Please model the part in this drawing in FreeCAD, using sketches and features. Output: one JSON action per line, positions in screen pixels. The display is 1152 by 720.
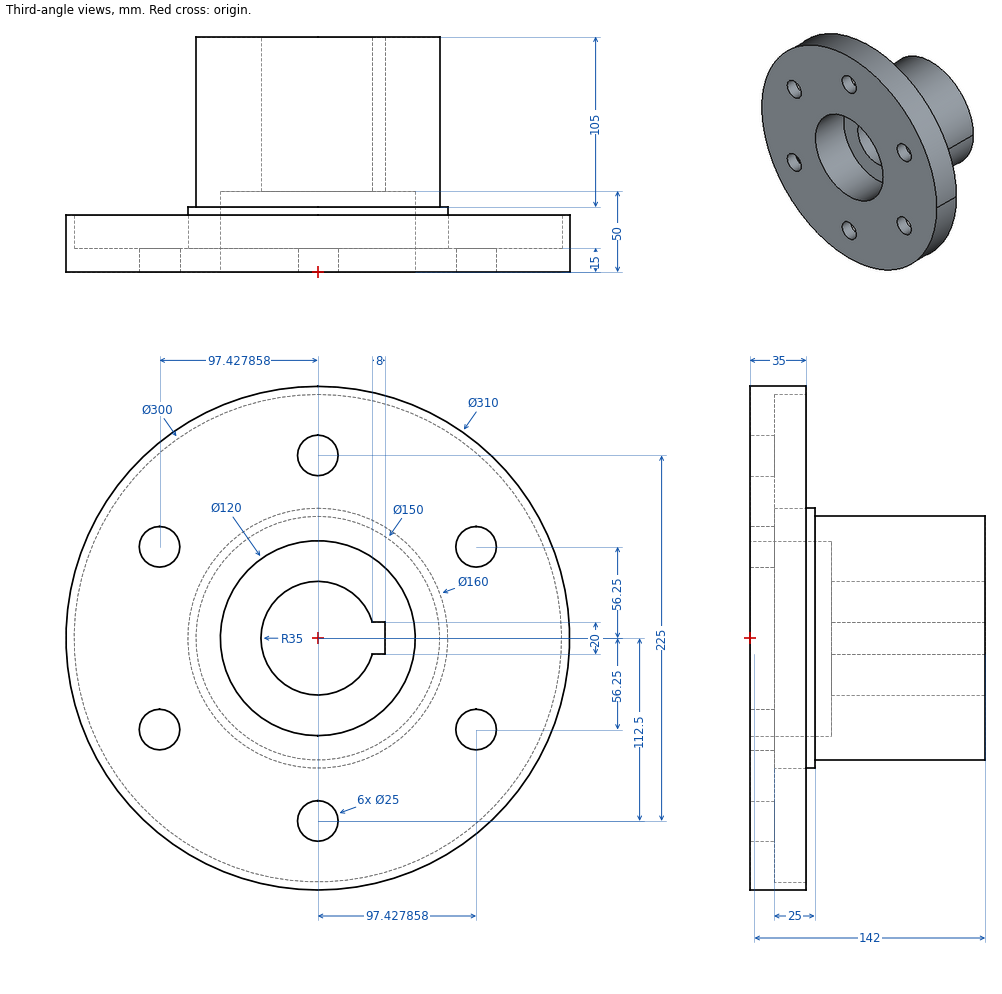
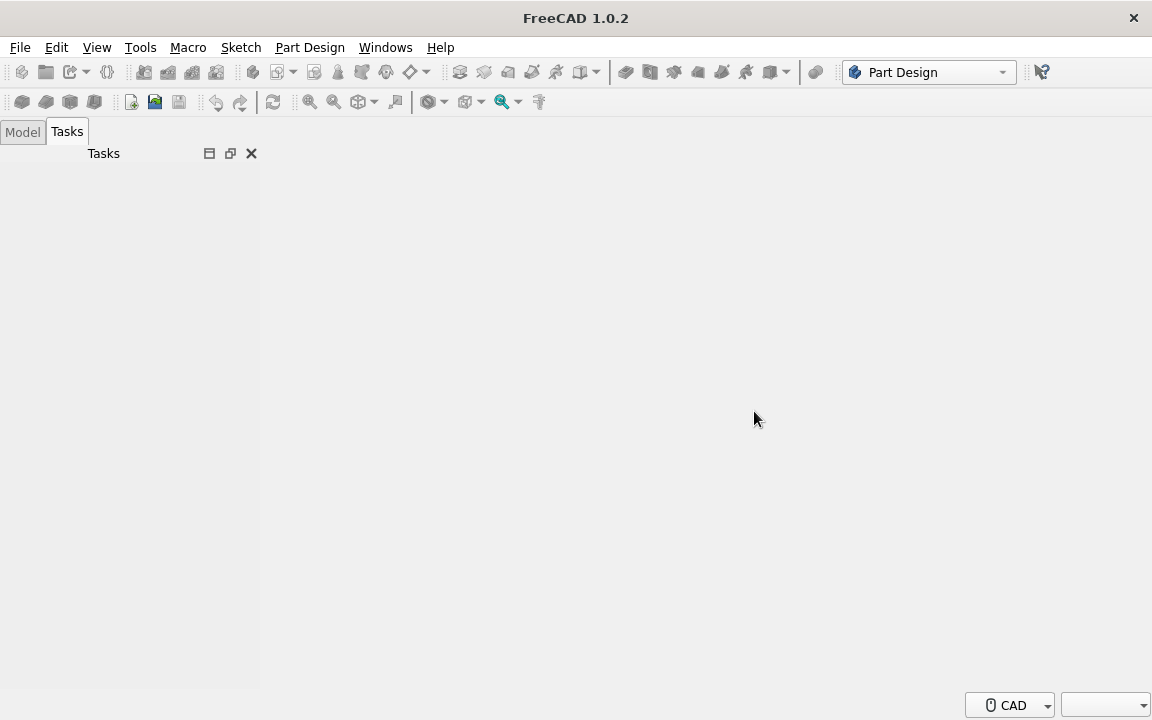
{"action": "left_click", "coordinate": [132, 102]}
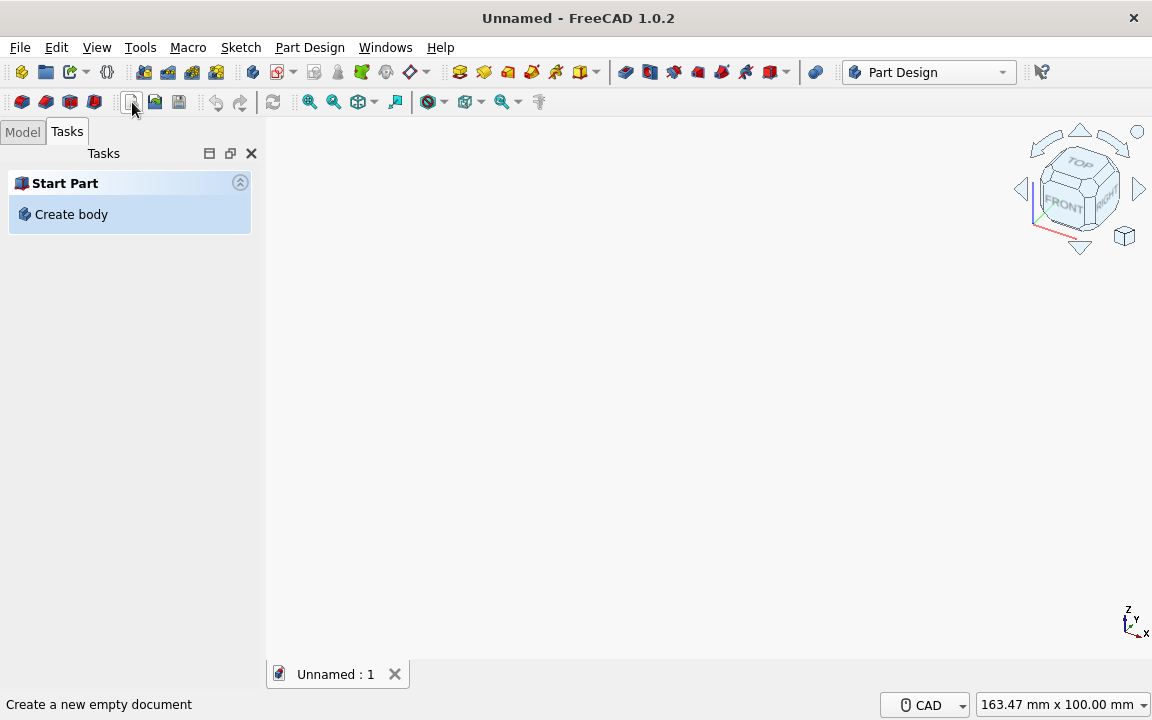
{"action": "left_click", "coordinate": [278, 72]}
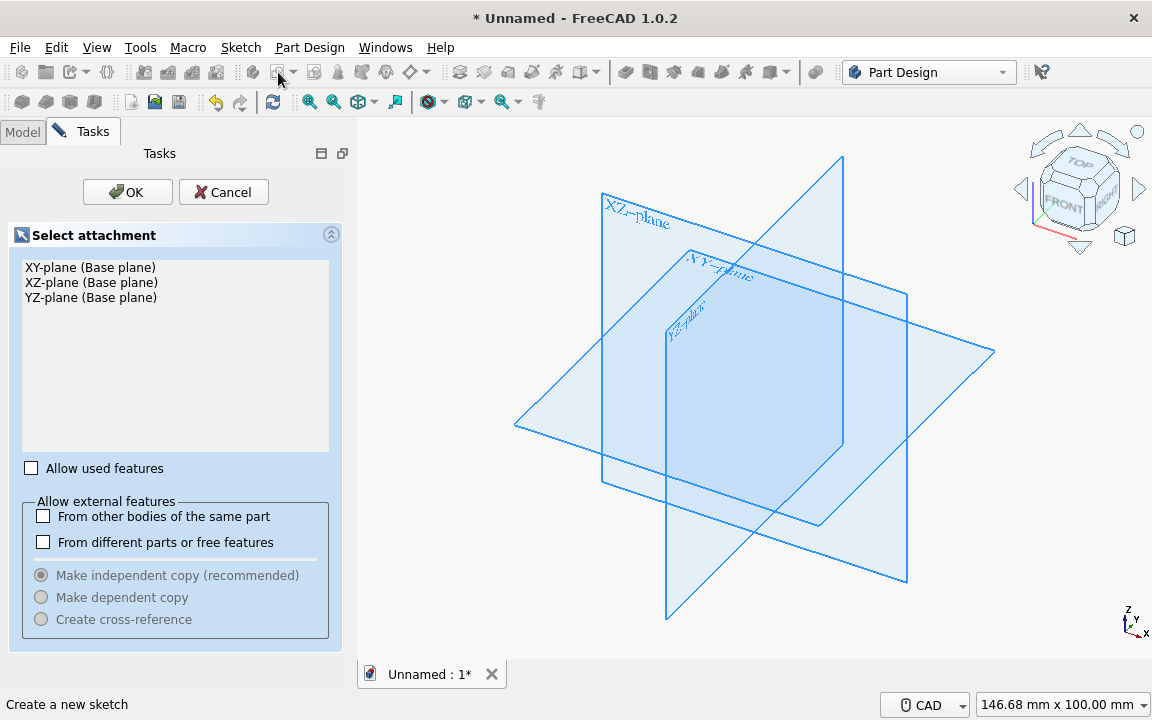
{"action": "left_click", "coordinate": [82, 282]}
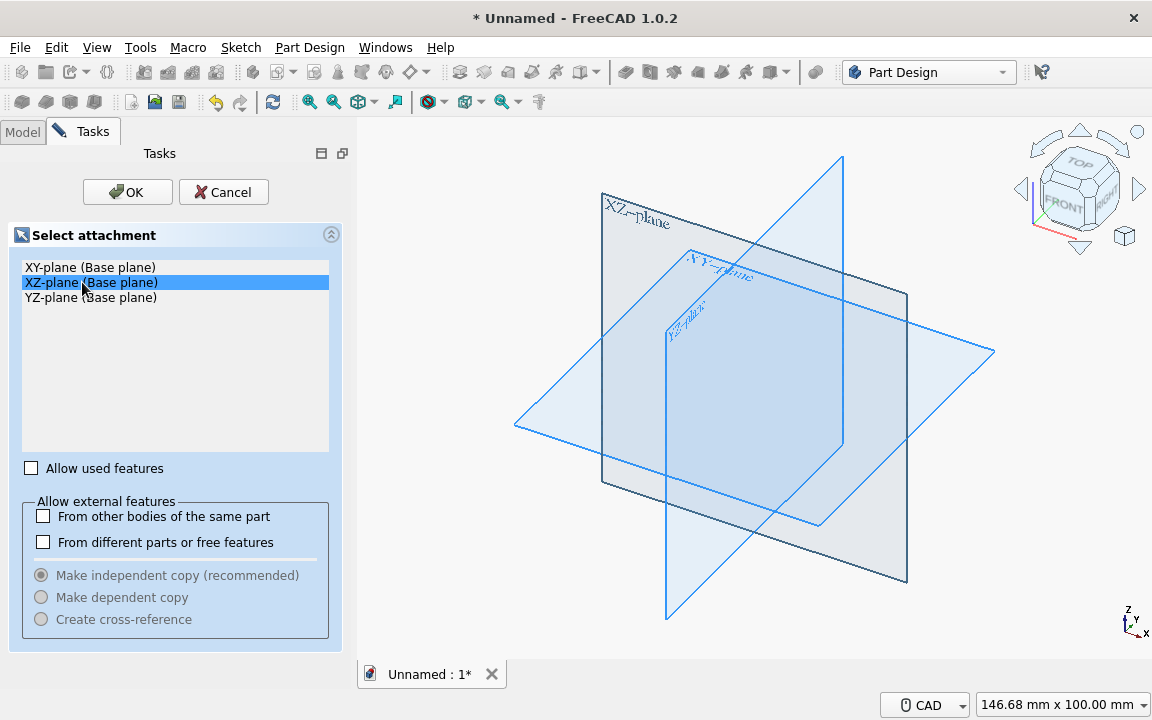
{"action": "left_click", "coordinate": [128, 192]}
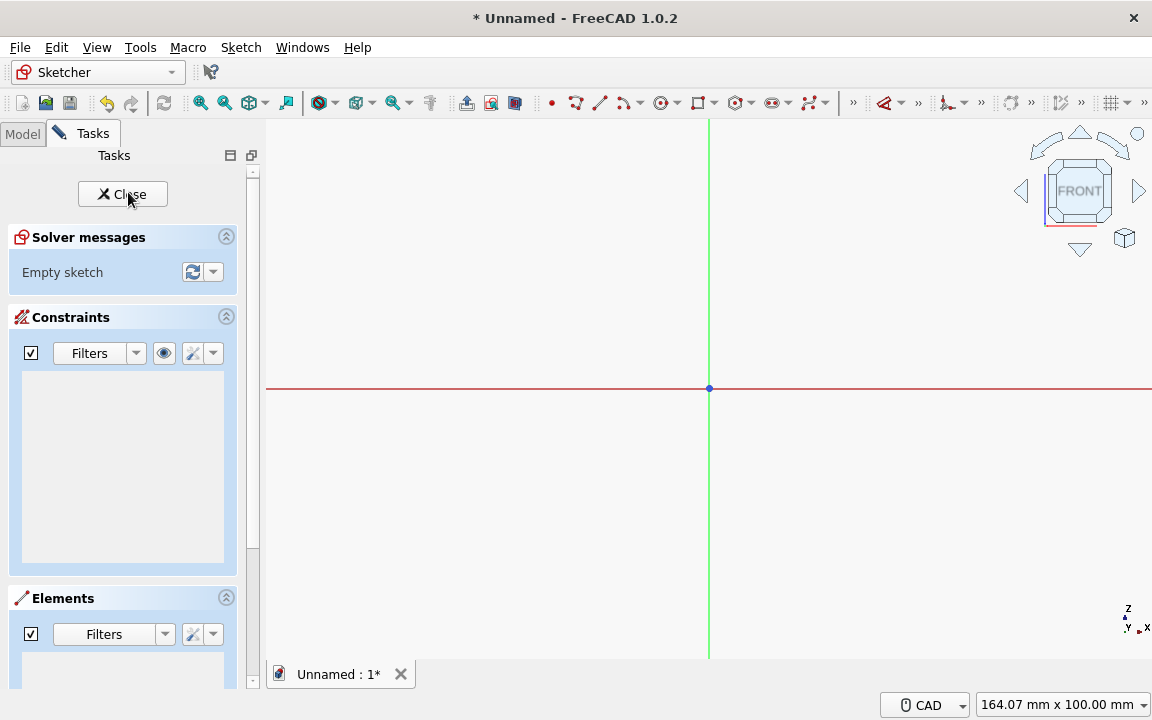
{"action": "scroll", "coordinate": [623, 389], "scroll_direction": "down", "scroll_amount": 8}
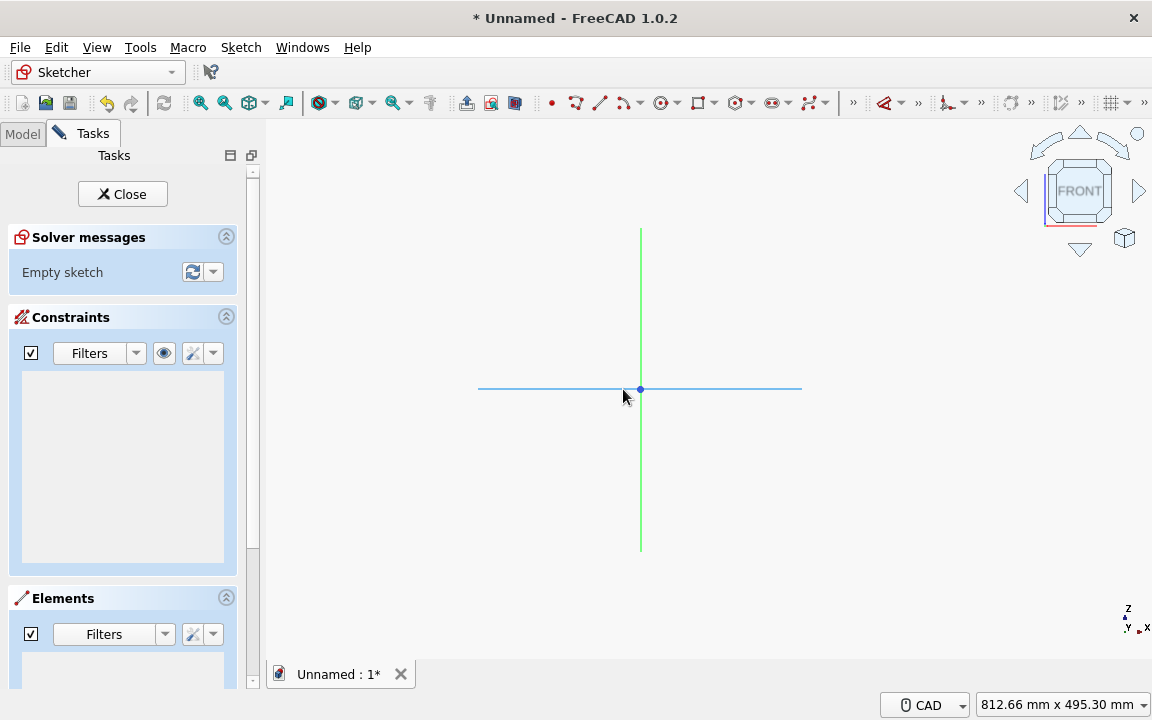
{"action": "left_click", "coordinate": [662, 104]}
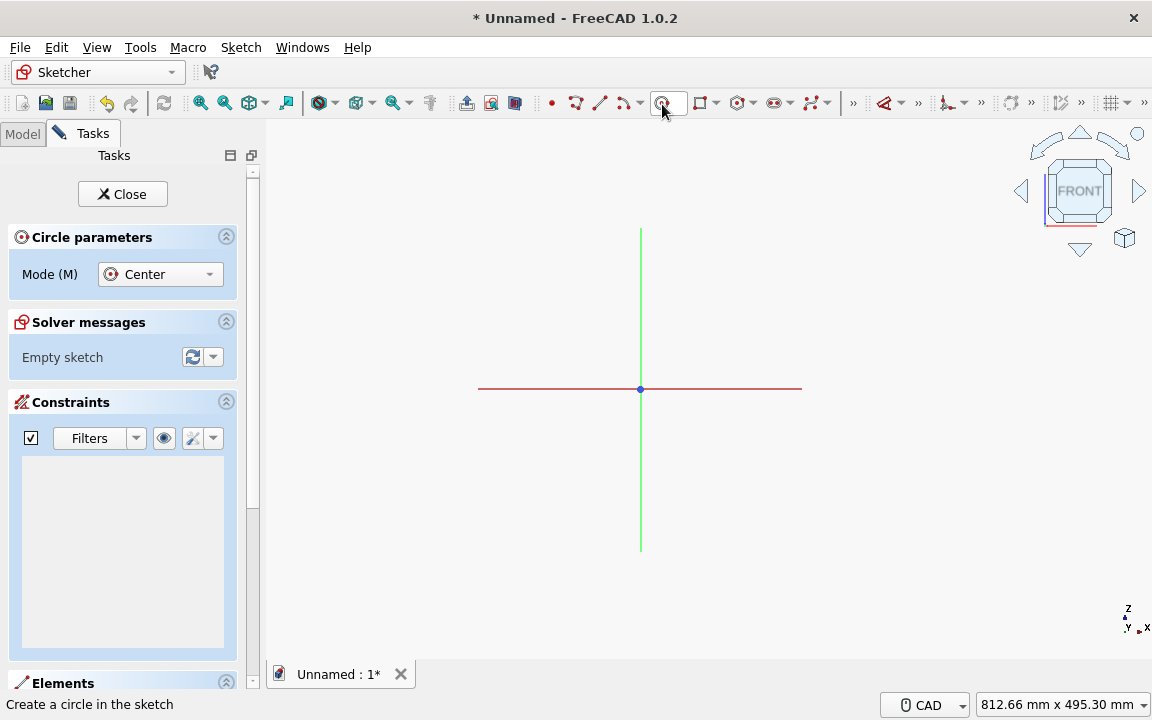
{"action": "left_click", "coordinate": [641, 389]}
{"action": "mouse_move", "coordinate": [760, 270]}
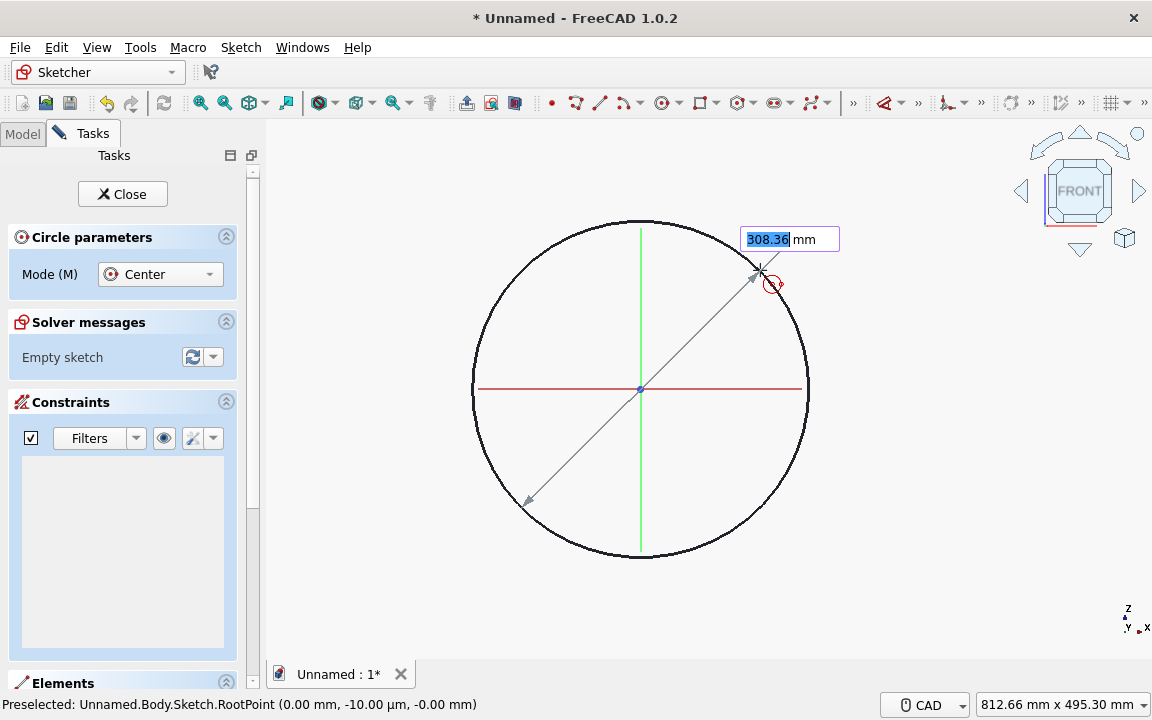
{"action": "type", "text": "310"}
{"action": "key", "text": "Return"}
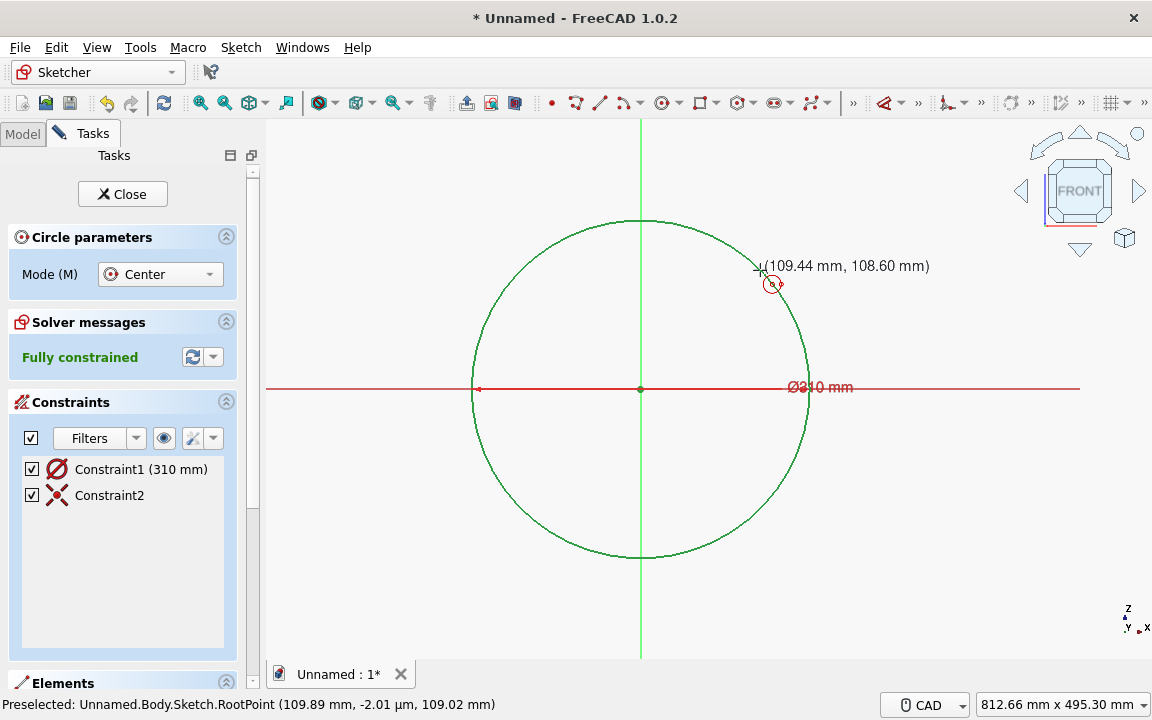
{"action": "left_click", "coordinate": [641, 389]}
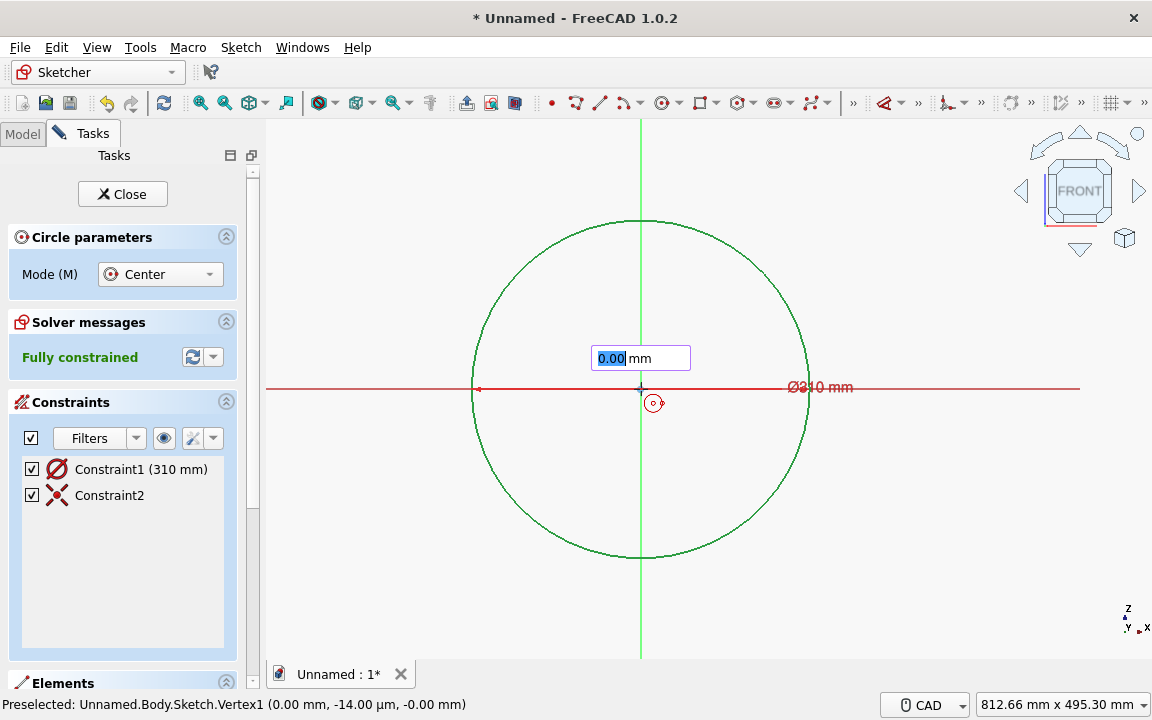
{"action": "scroll", "coordinate": [756, 274], "scroll_direction": "up", "scroll_amount": 6}
{"action": "mouse_move", "coordinate": [756, 273]}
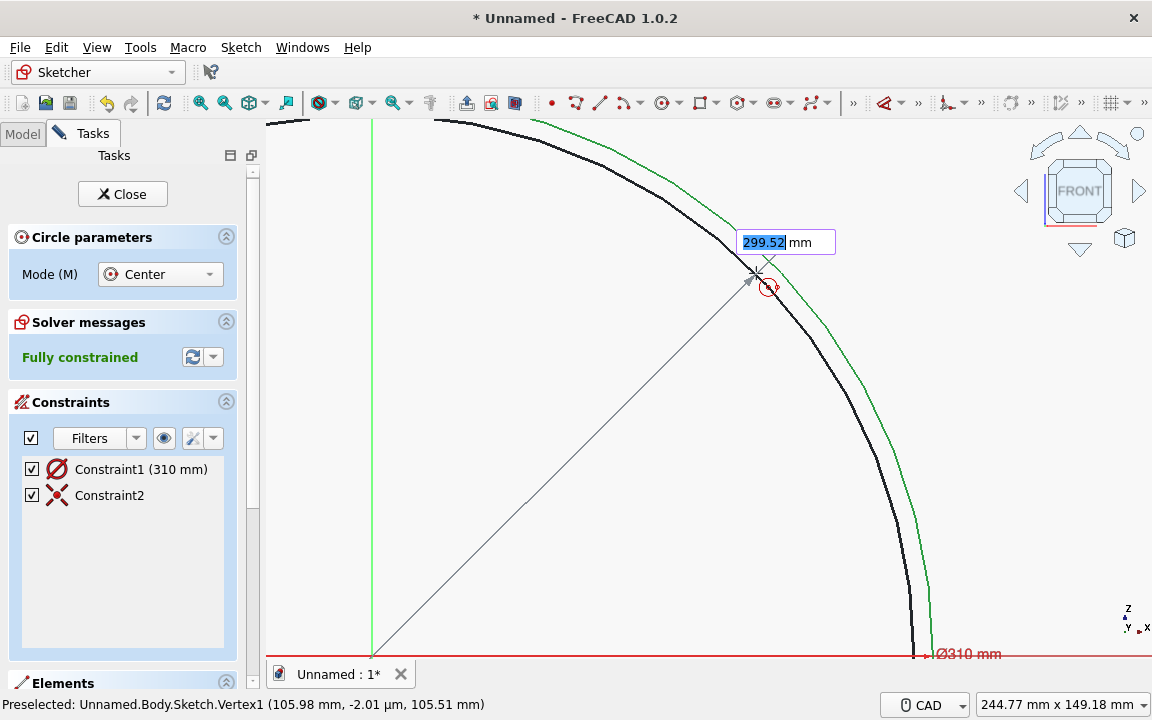
{"action": "type", "text": "300"}
{"action": "key", "text": "Return"}
{"action": "key", "text": "Escape"}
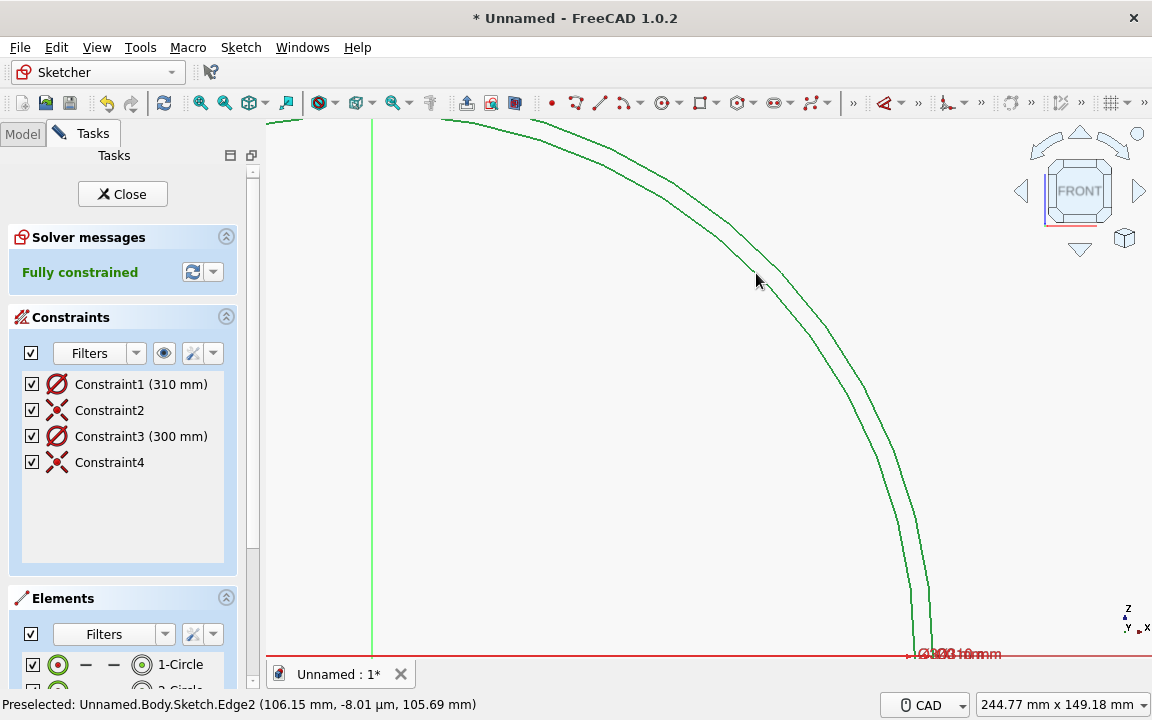
{"action": "left_click", "coordinate": [123, 194]}